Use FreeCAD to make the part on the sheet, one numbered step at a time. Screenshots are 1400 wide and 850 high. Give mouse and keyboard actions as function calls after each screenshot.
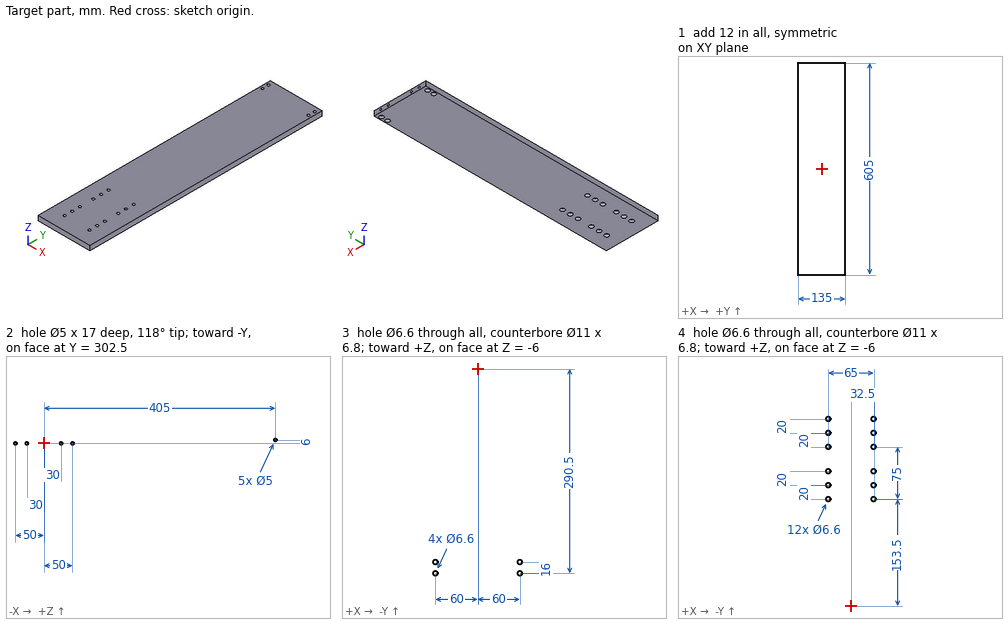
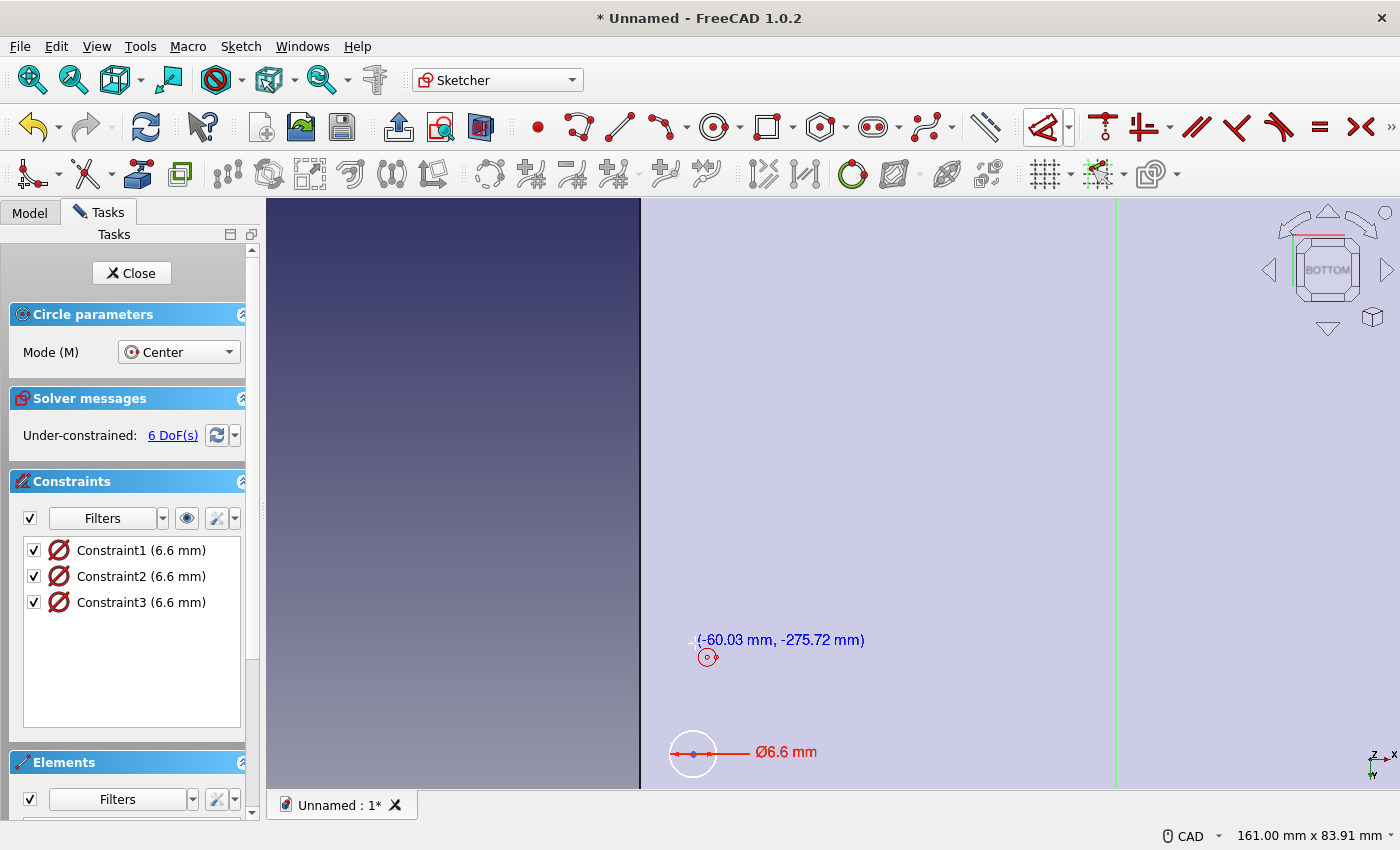
scroll(695, 643, down, 9)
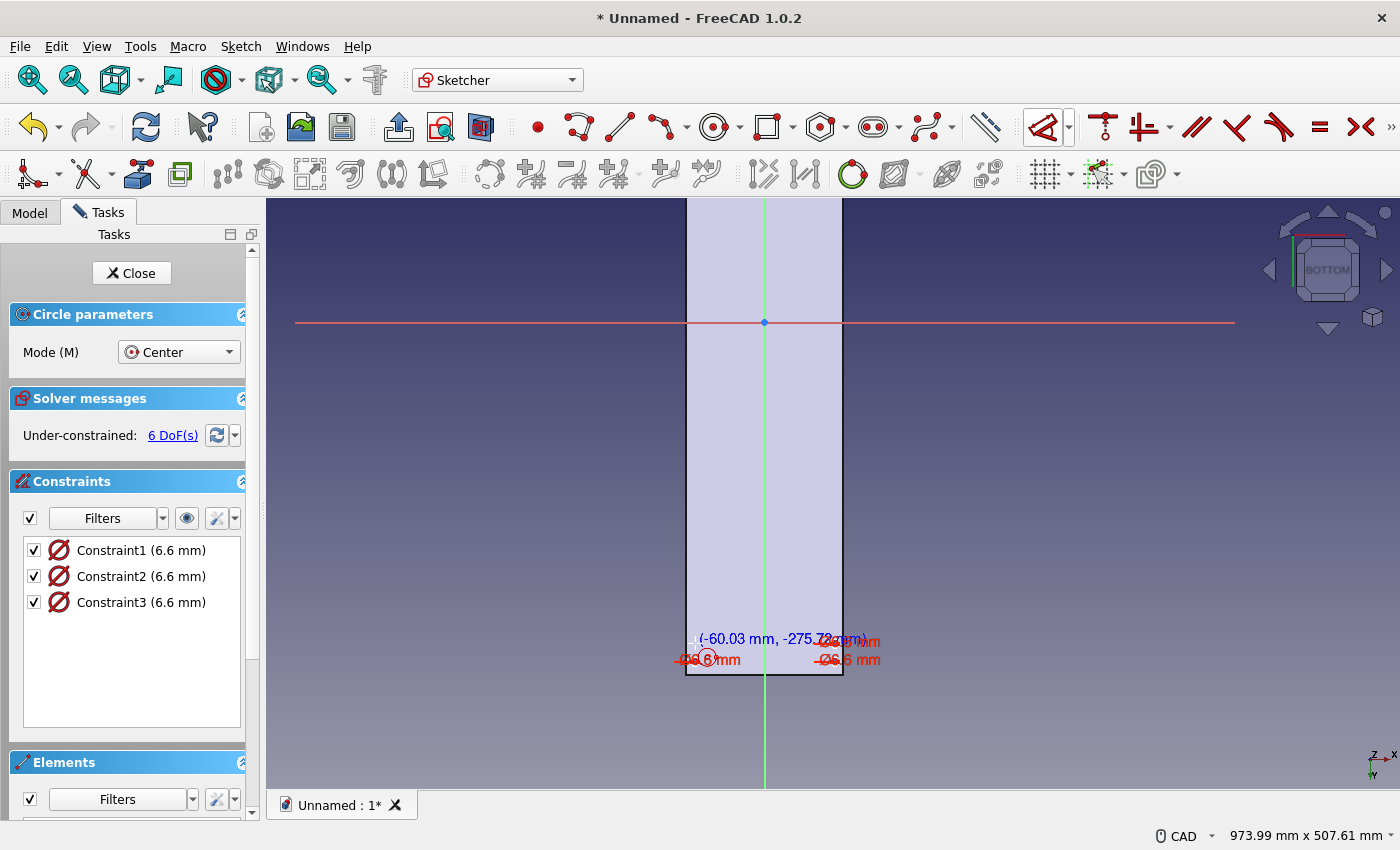
click(695, 643)
move(698, 640)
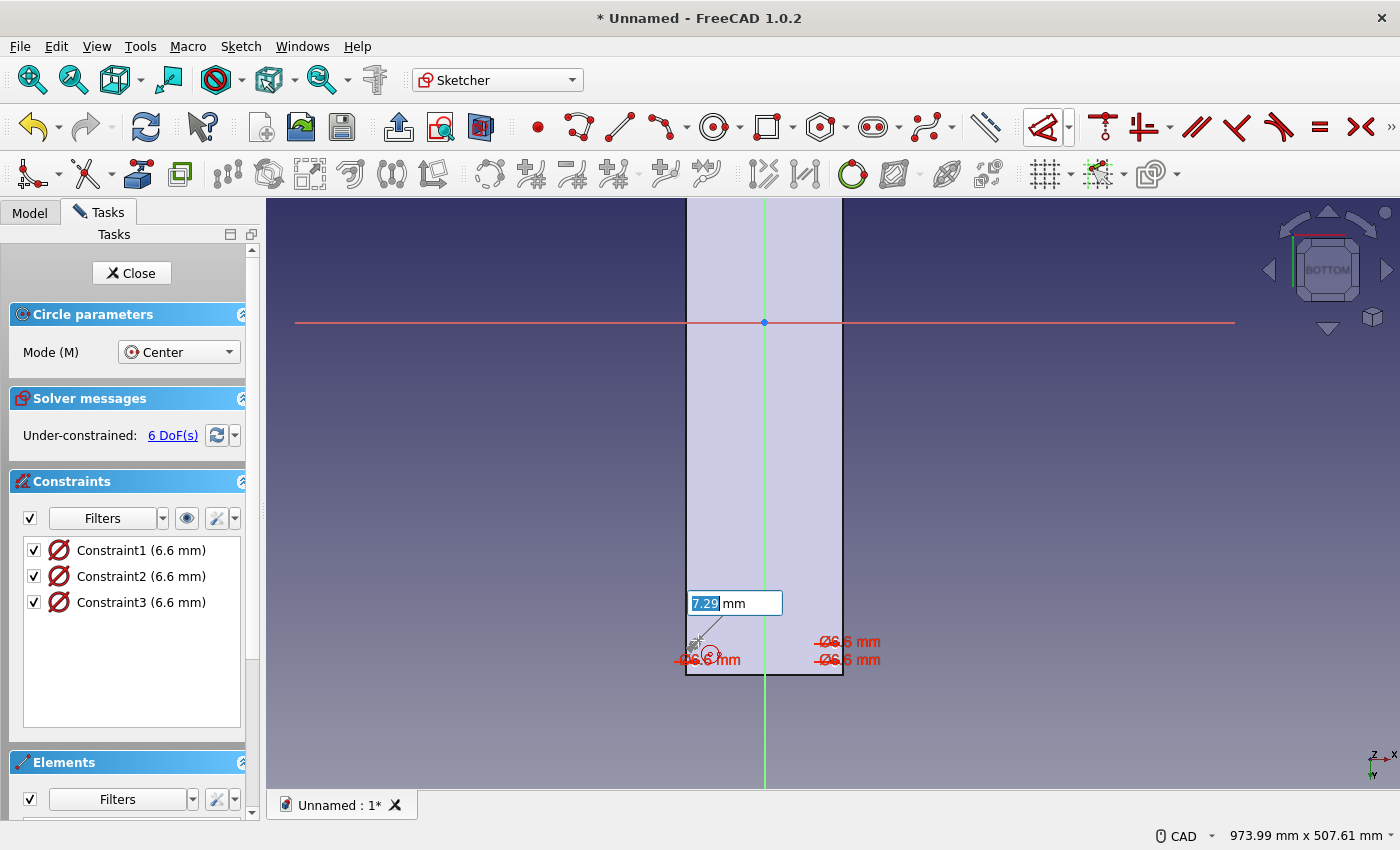
text(6.6)
key(Return)
key(Escape)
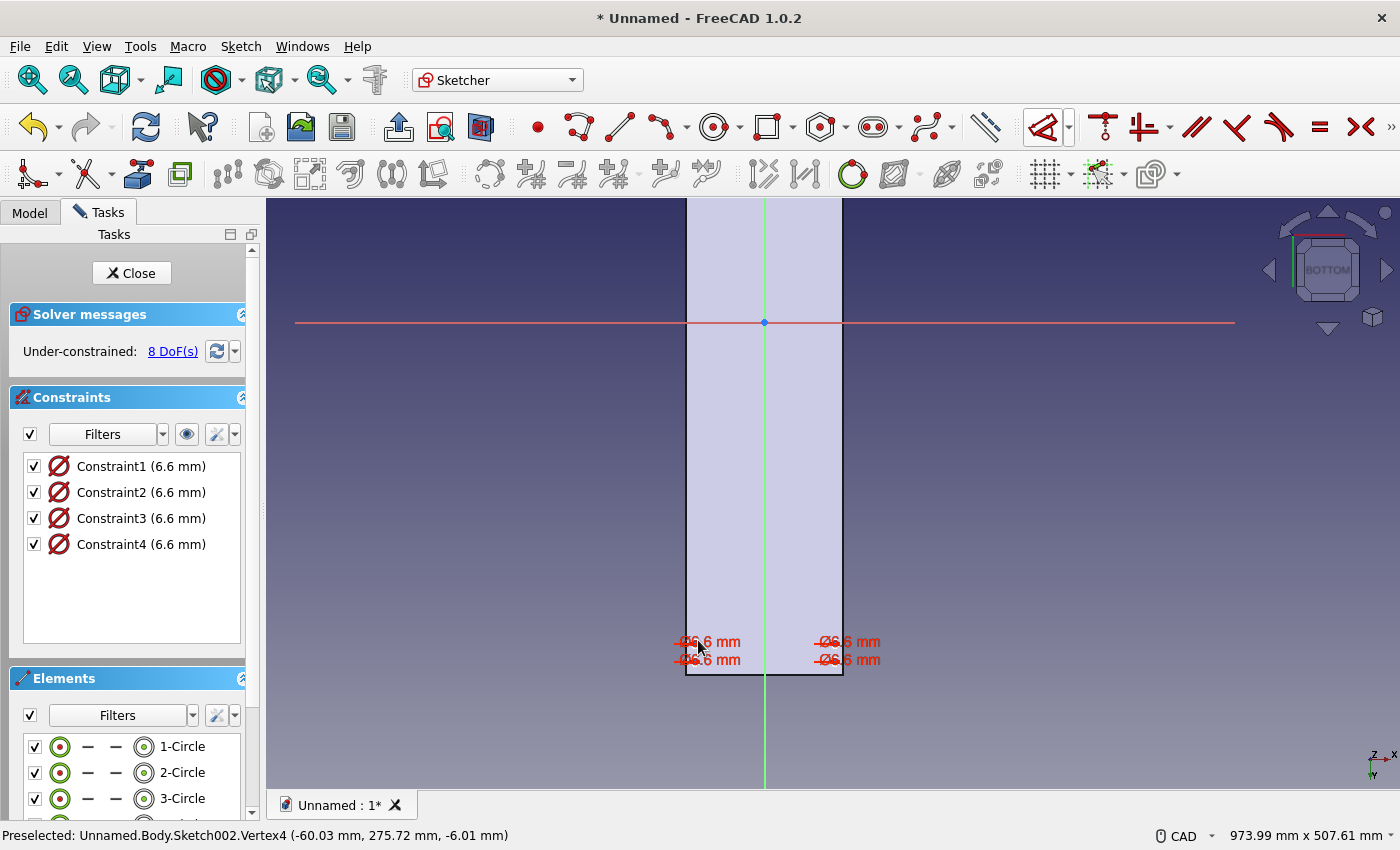
click(835, 662)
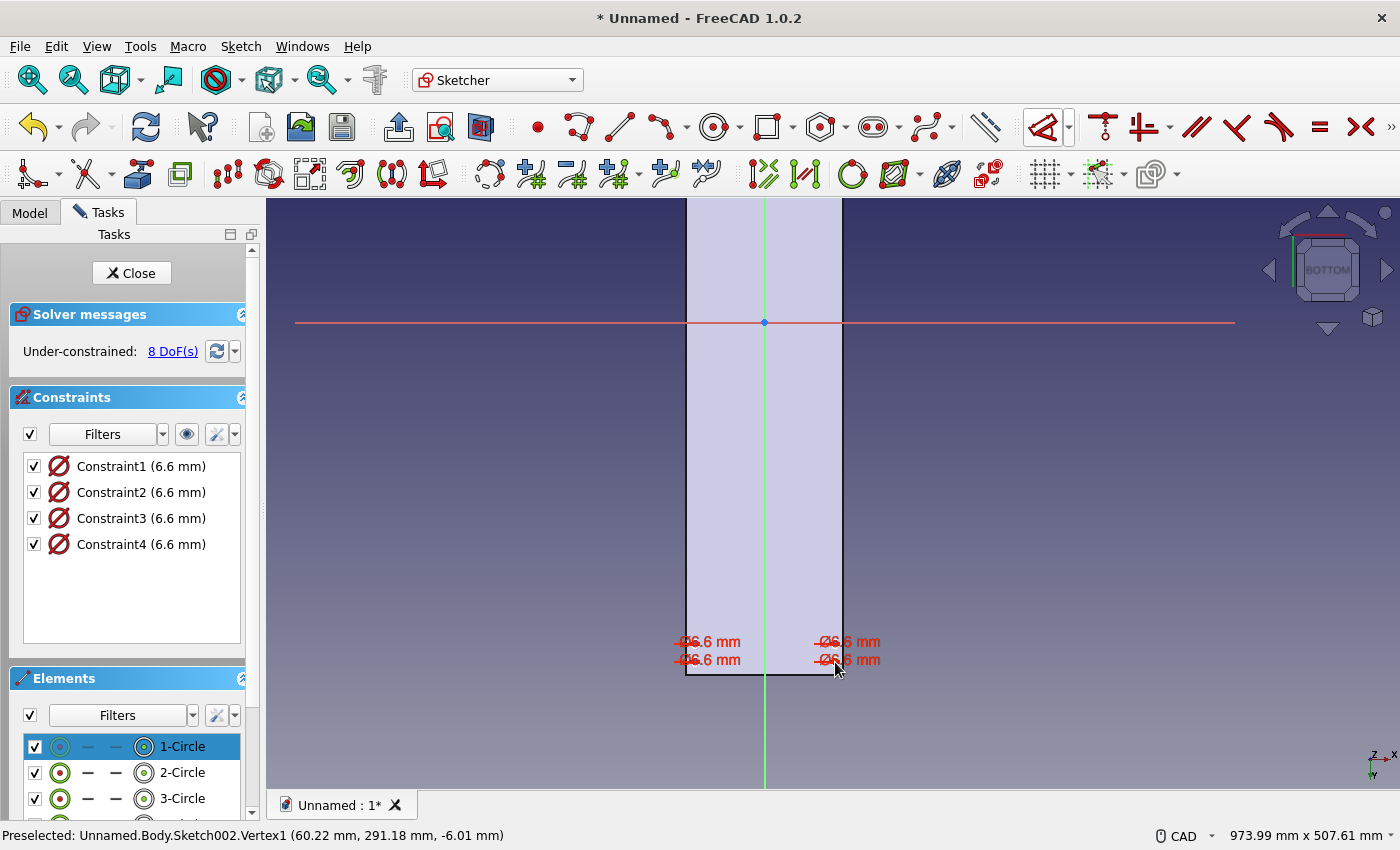
click(695, 662)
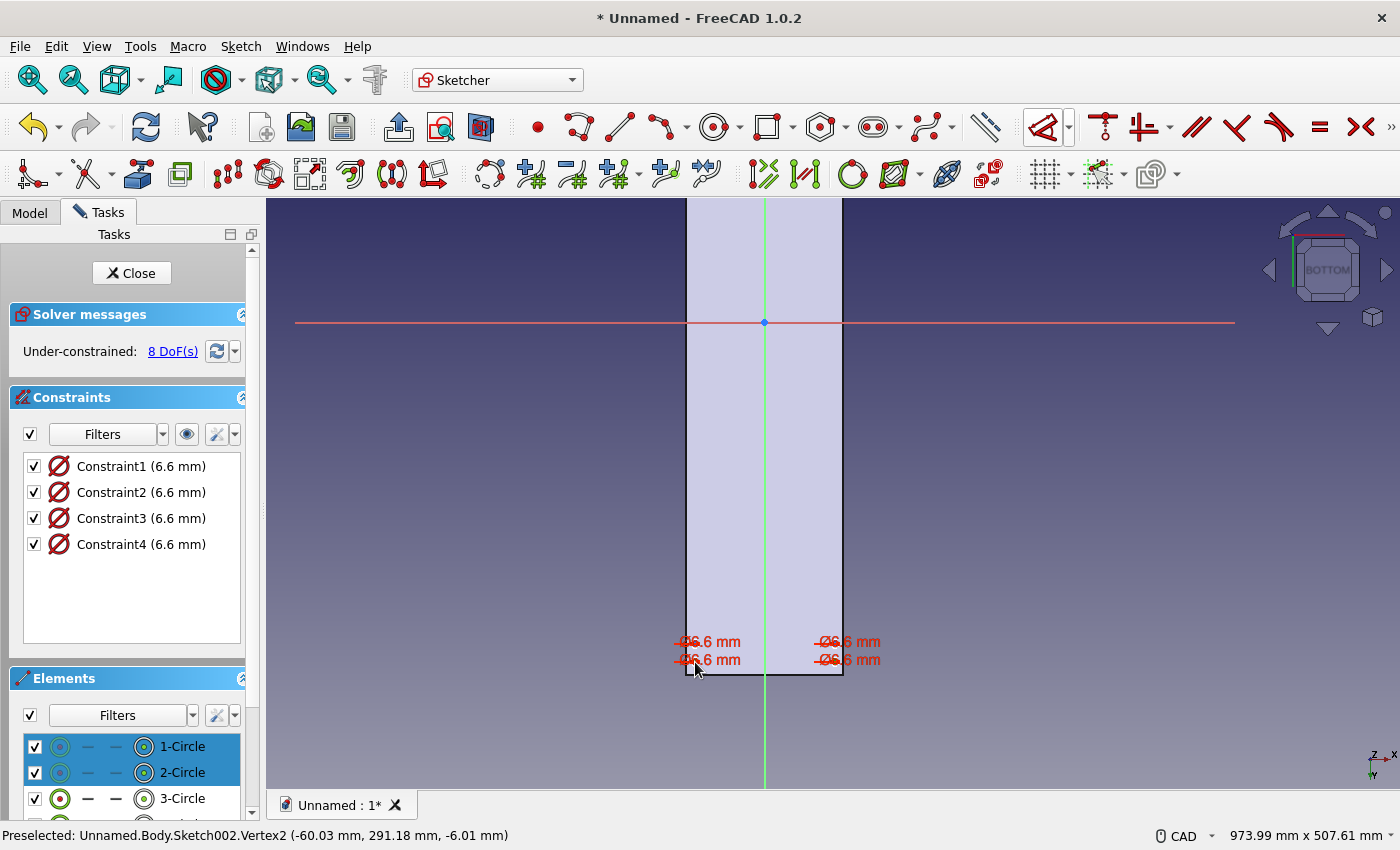
click(1170, 128)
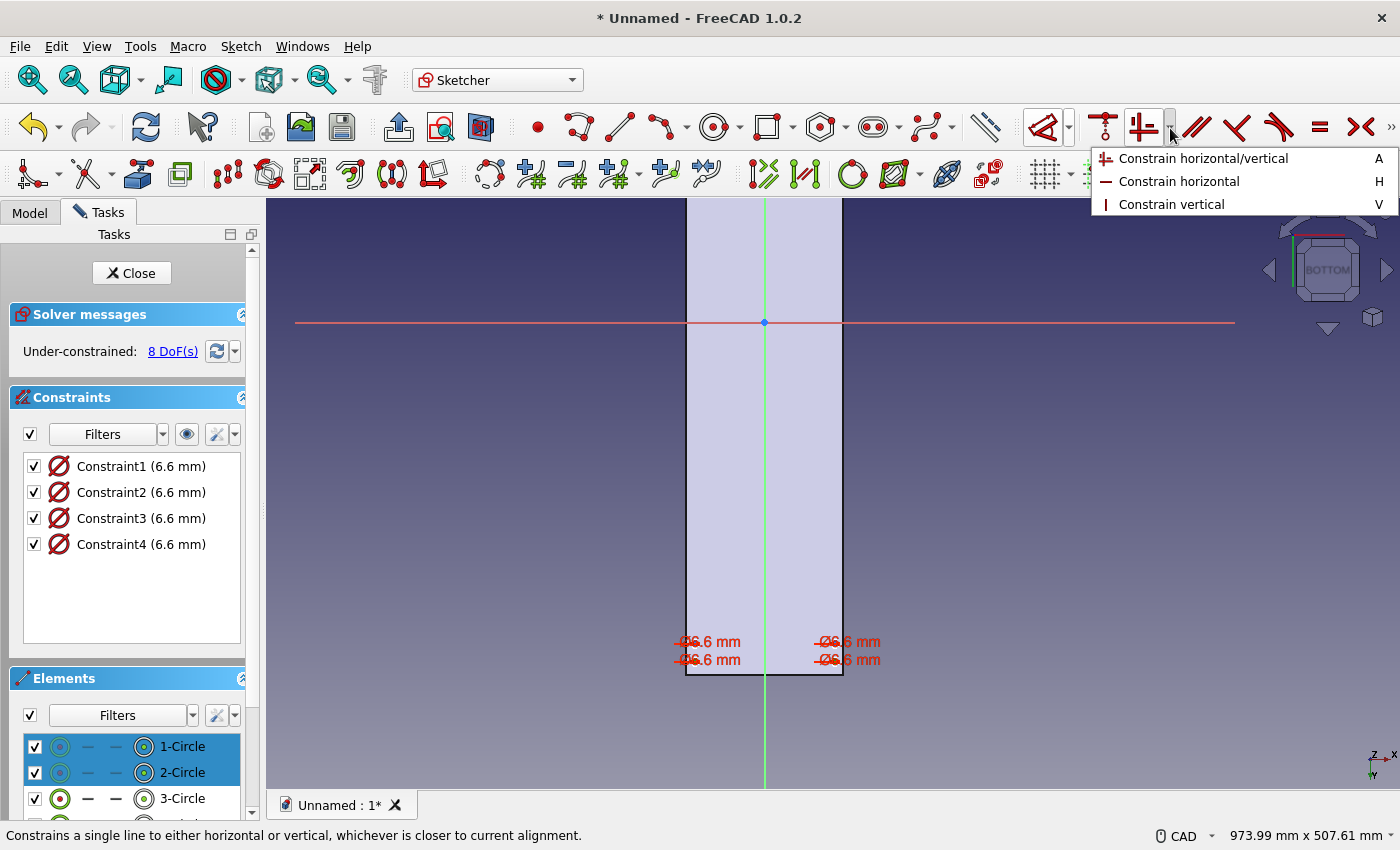
click(1245, 182)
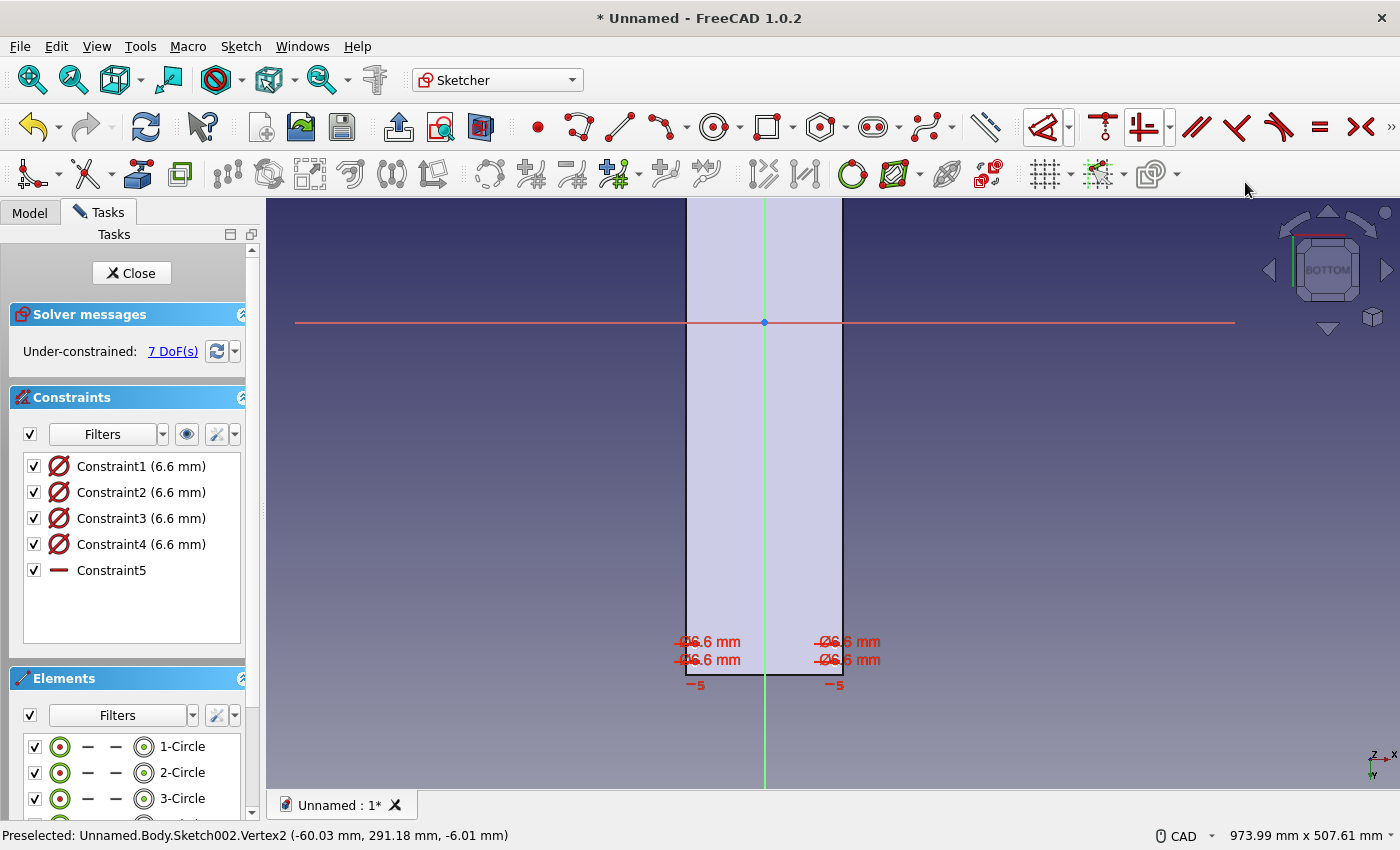
click(835, 662)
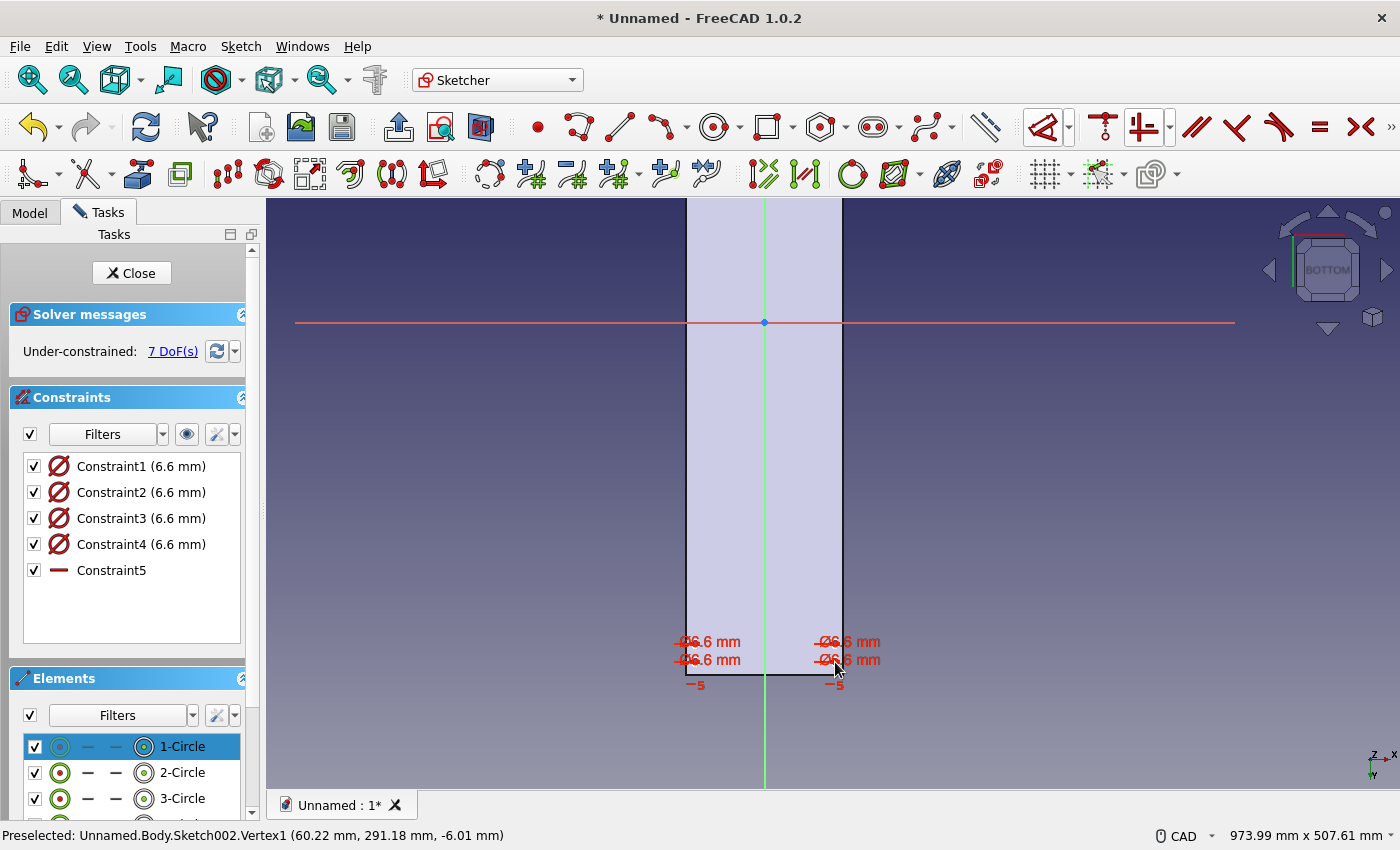
click(835, 644)